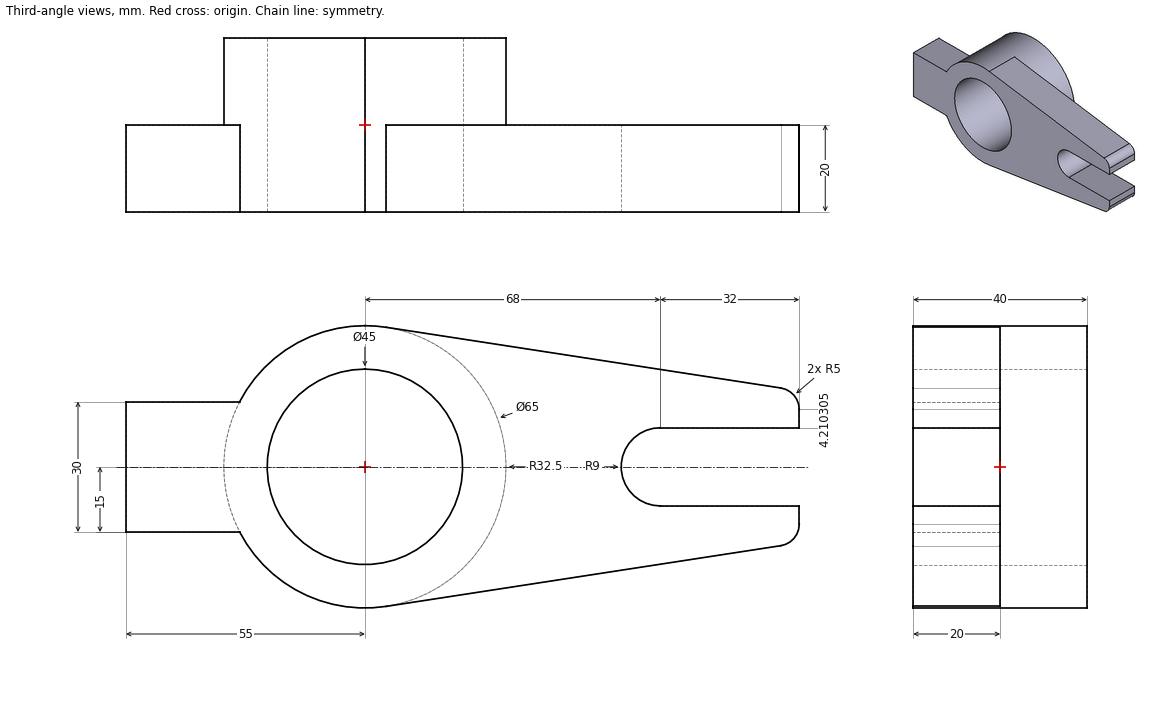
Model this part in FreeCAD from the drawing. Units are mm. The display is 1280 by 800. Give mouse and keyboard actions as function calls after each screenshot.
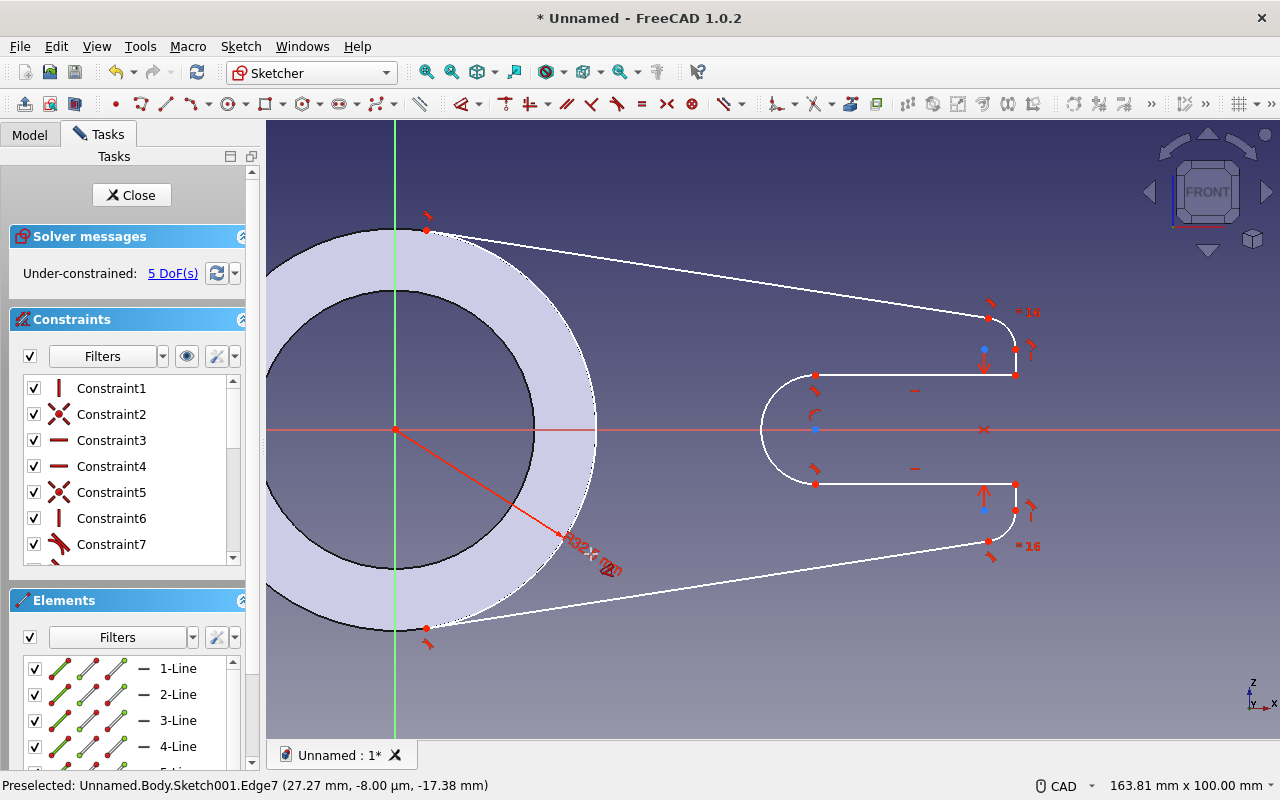
scroll(1013, 336, up, 2)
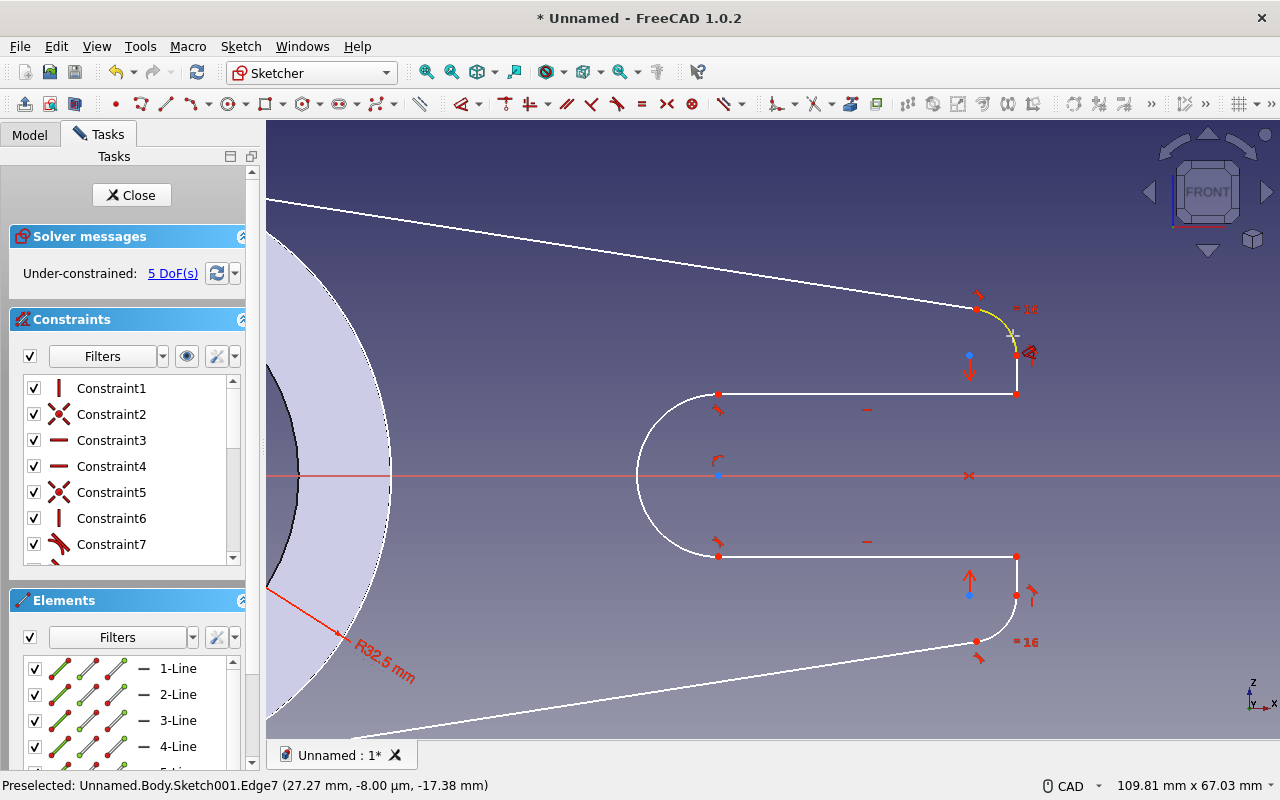
click(1012, 336)
click(1041, 323)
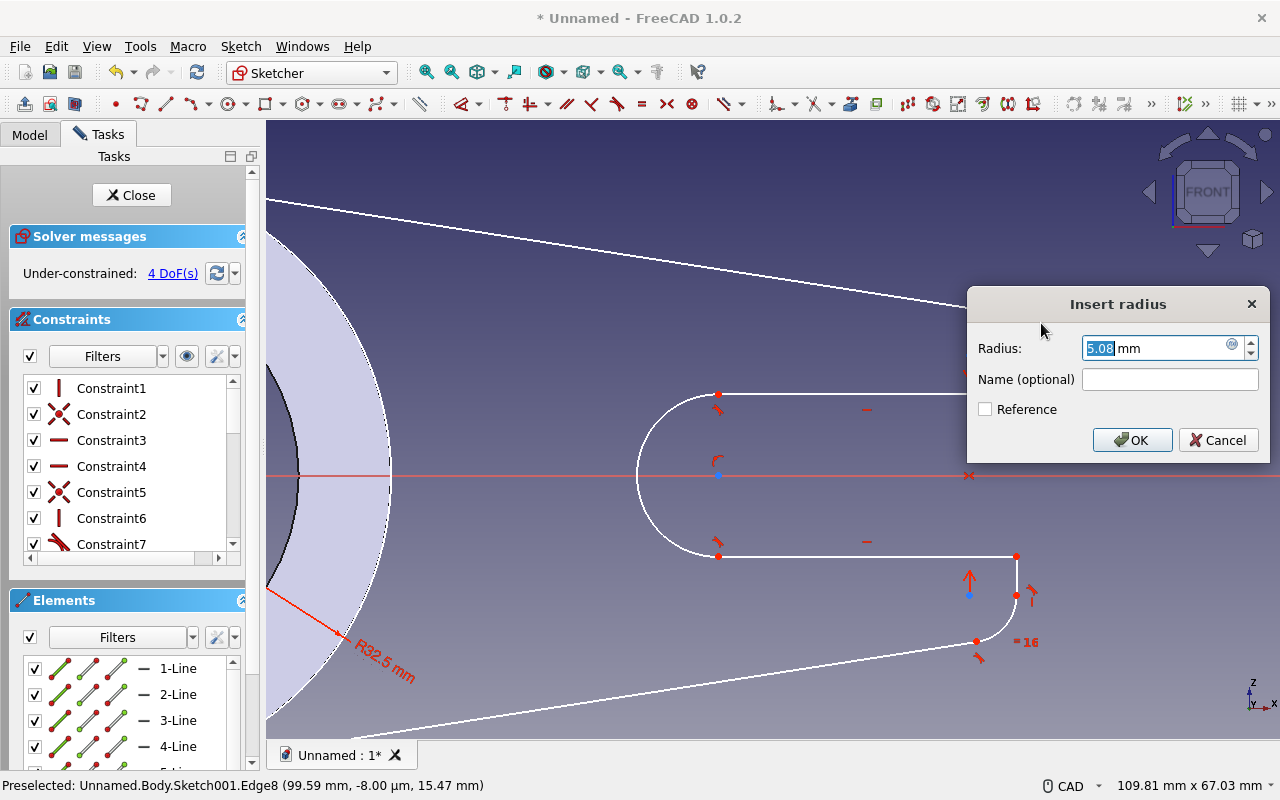
text(5)
key(Return)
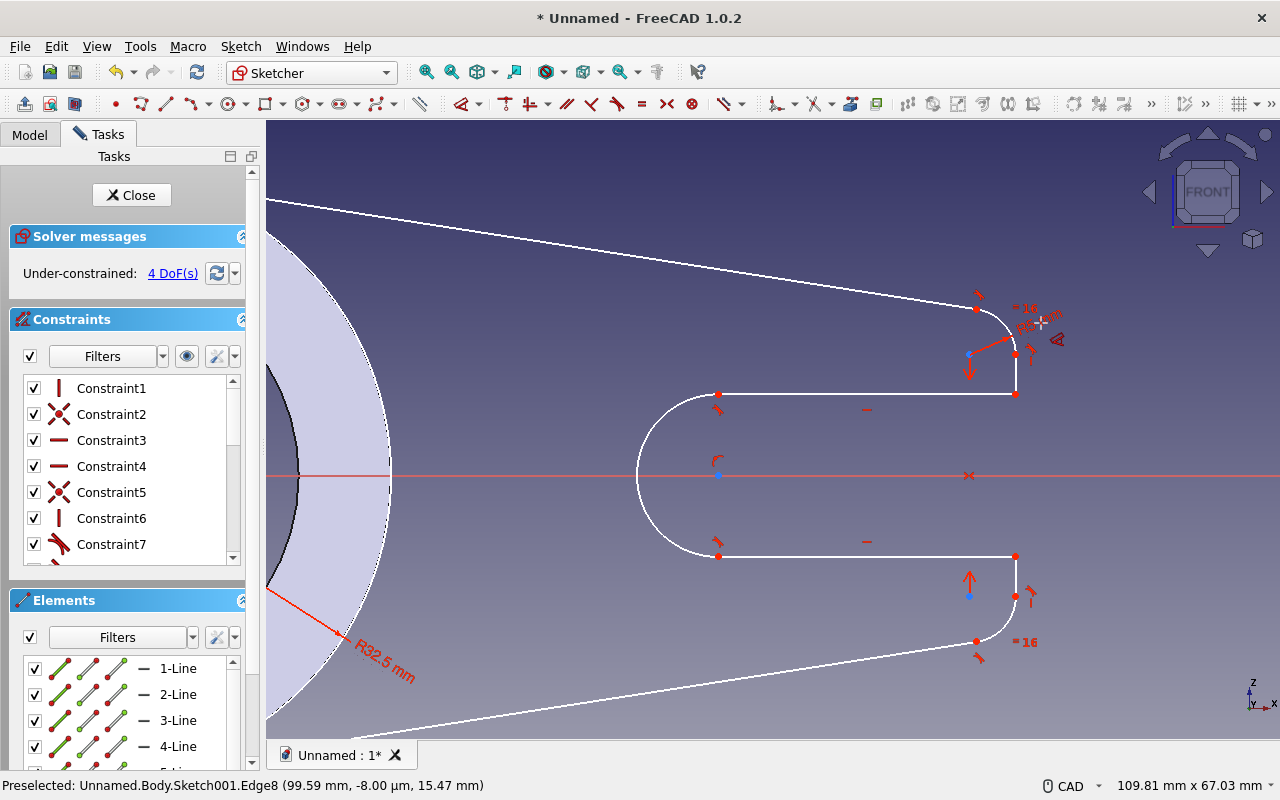
click(653, 428)
click(627, 409)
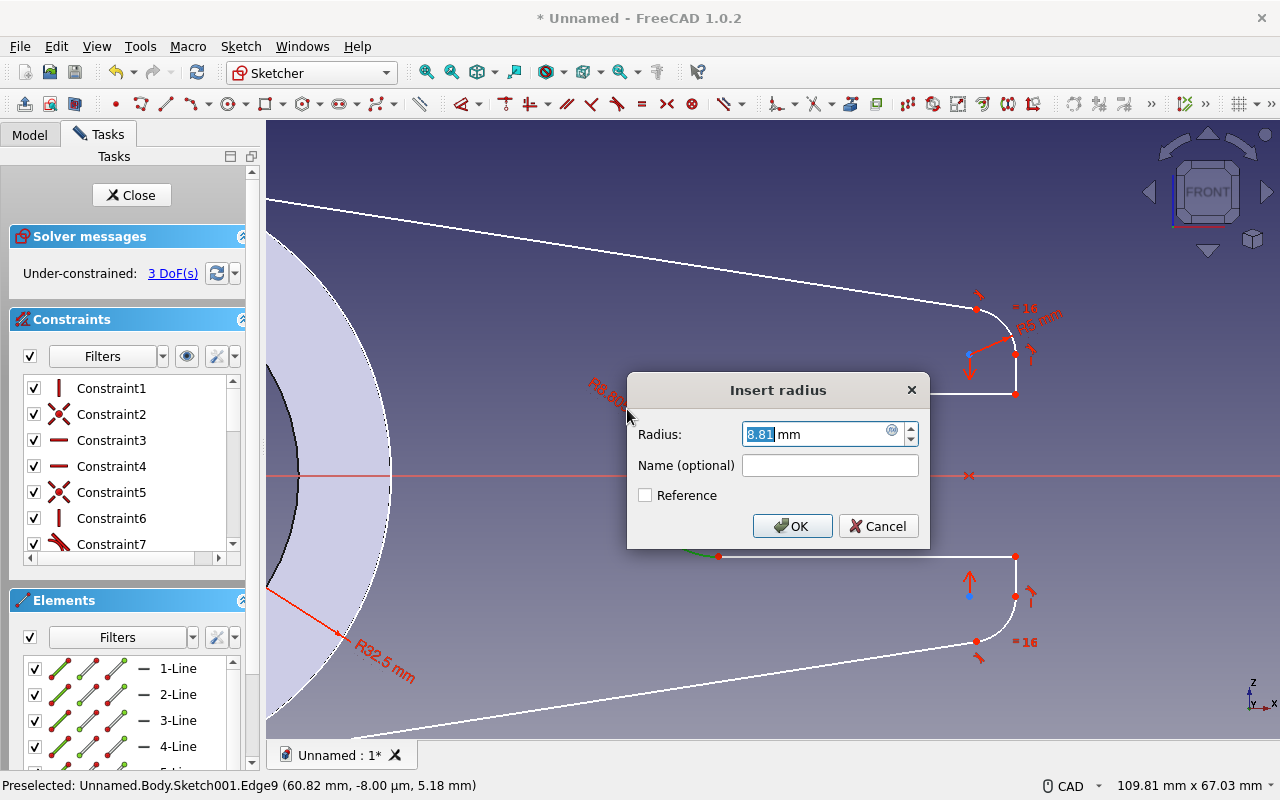
text(9)
key(Return)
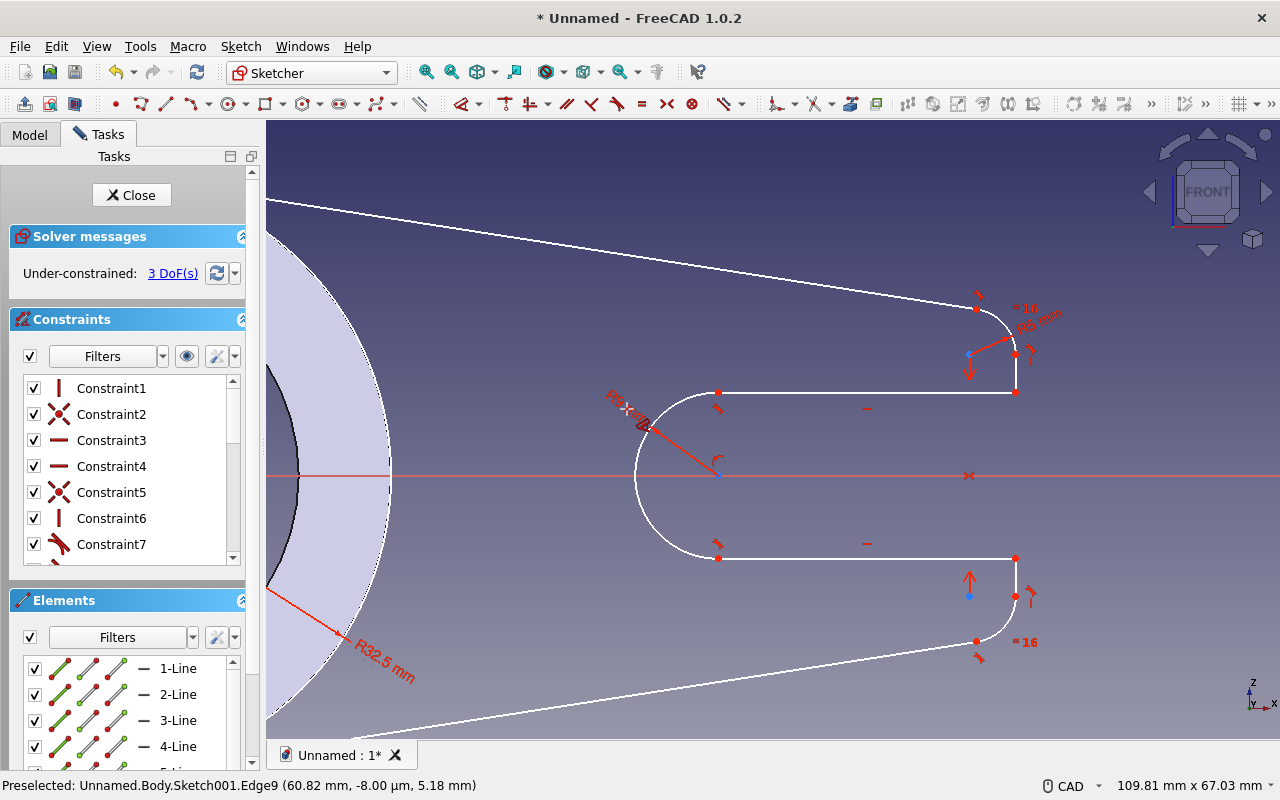
click(927, 393)
click(867, 359)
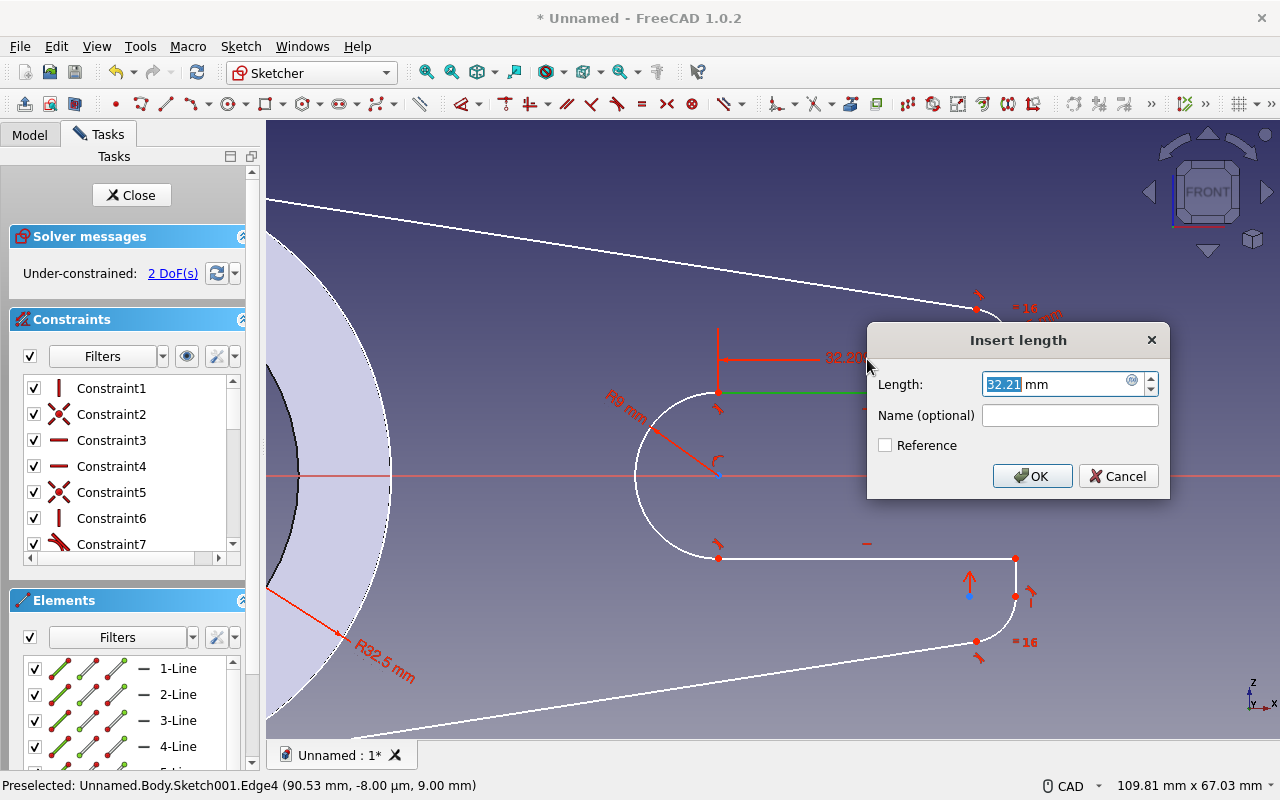
text(32)
key(Return)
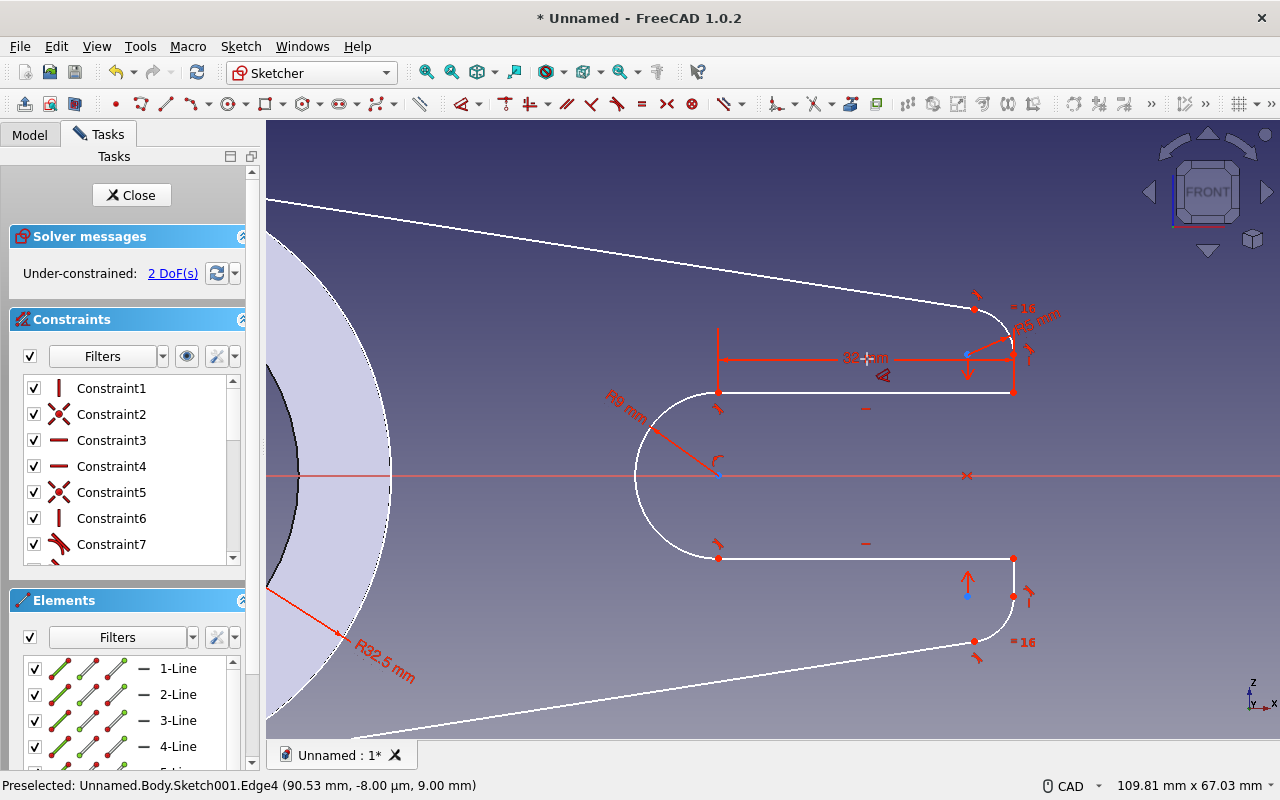
click(718, 393)
click(506, 359)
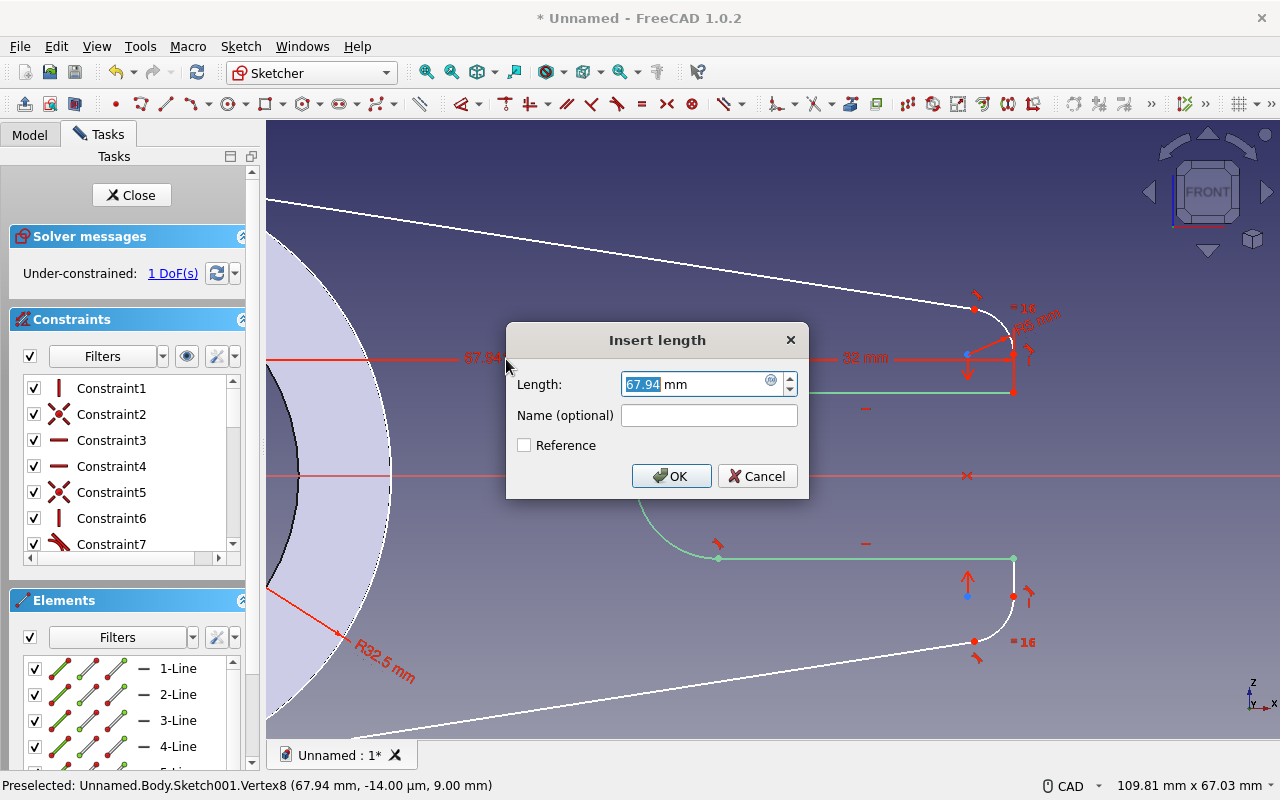
text(68)
key(Return)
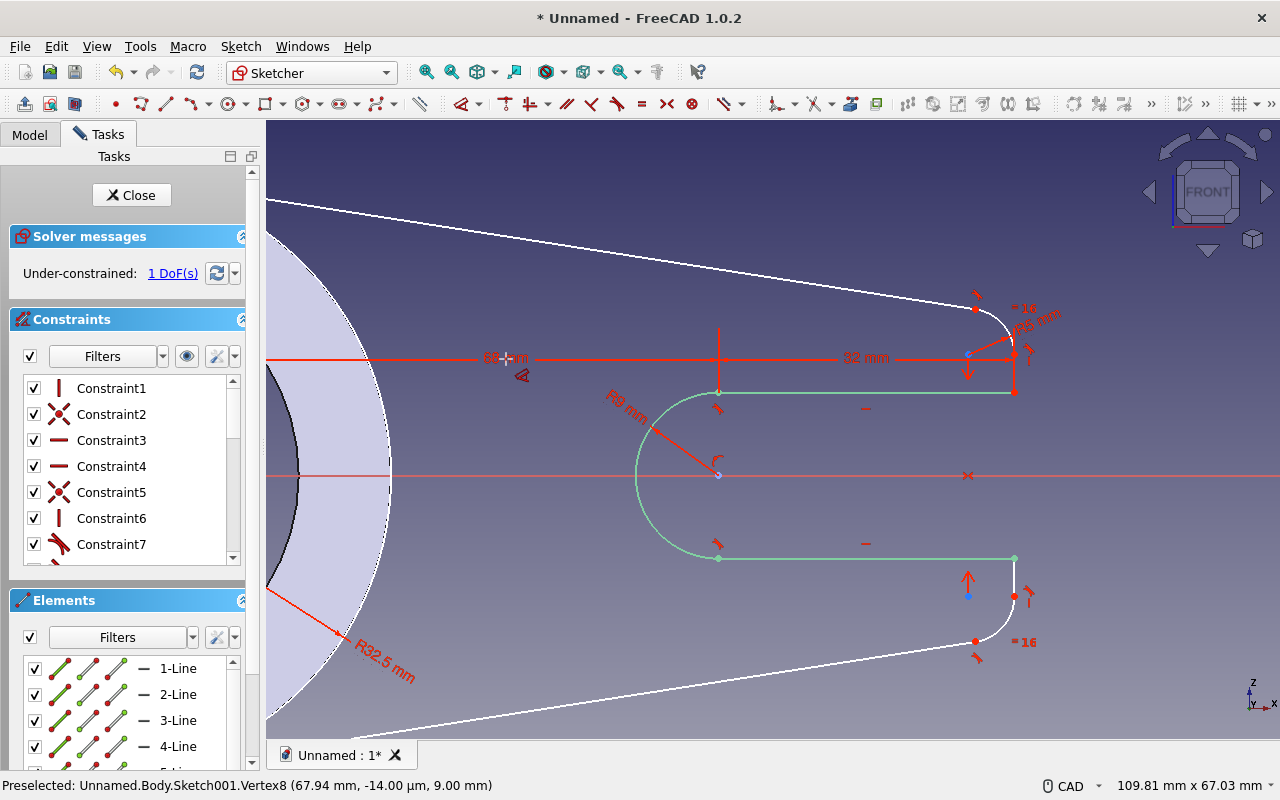
scroll(1014, 366, up, 2)